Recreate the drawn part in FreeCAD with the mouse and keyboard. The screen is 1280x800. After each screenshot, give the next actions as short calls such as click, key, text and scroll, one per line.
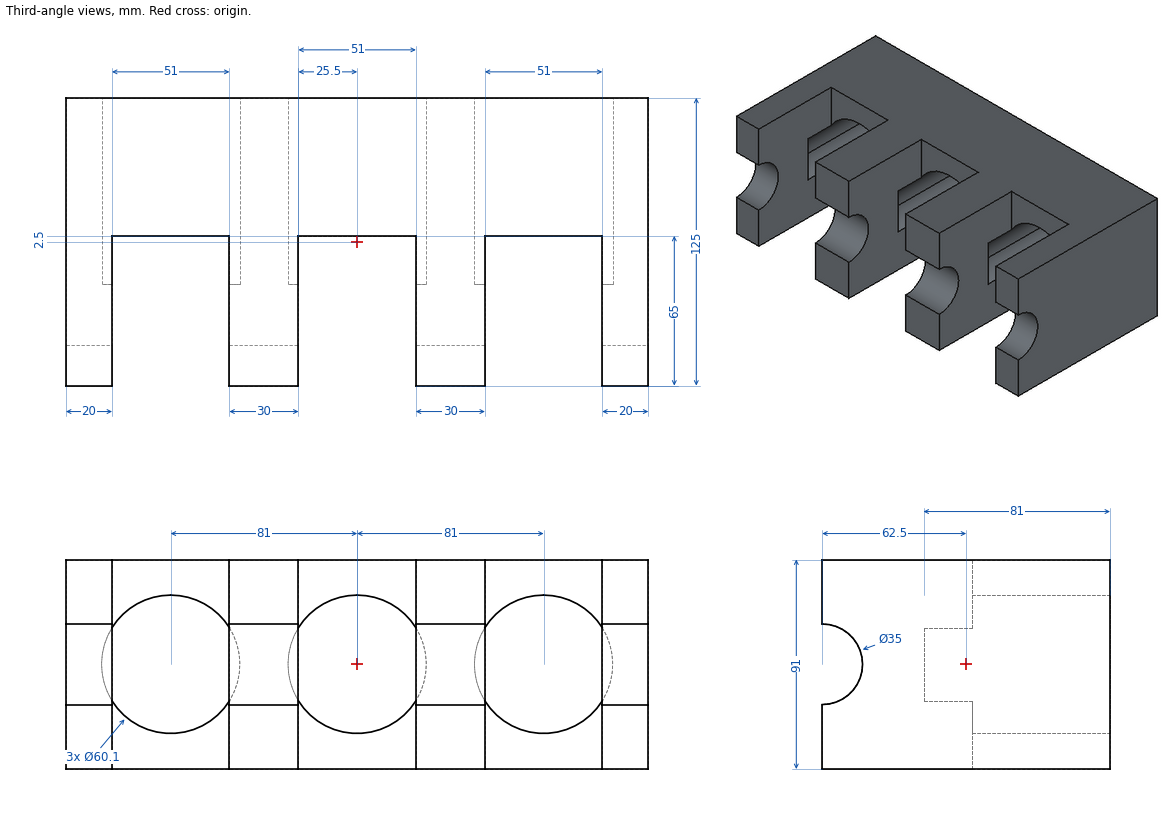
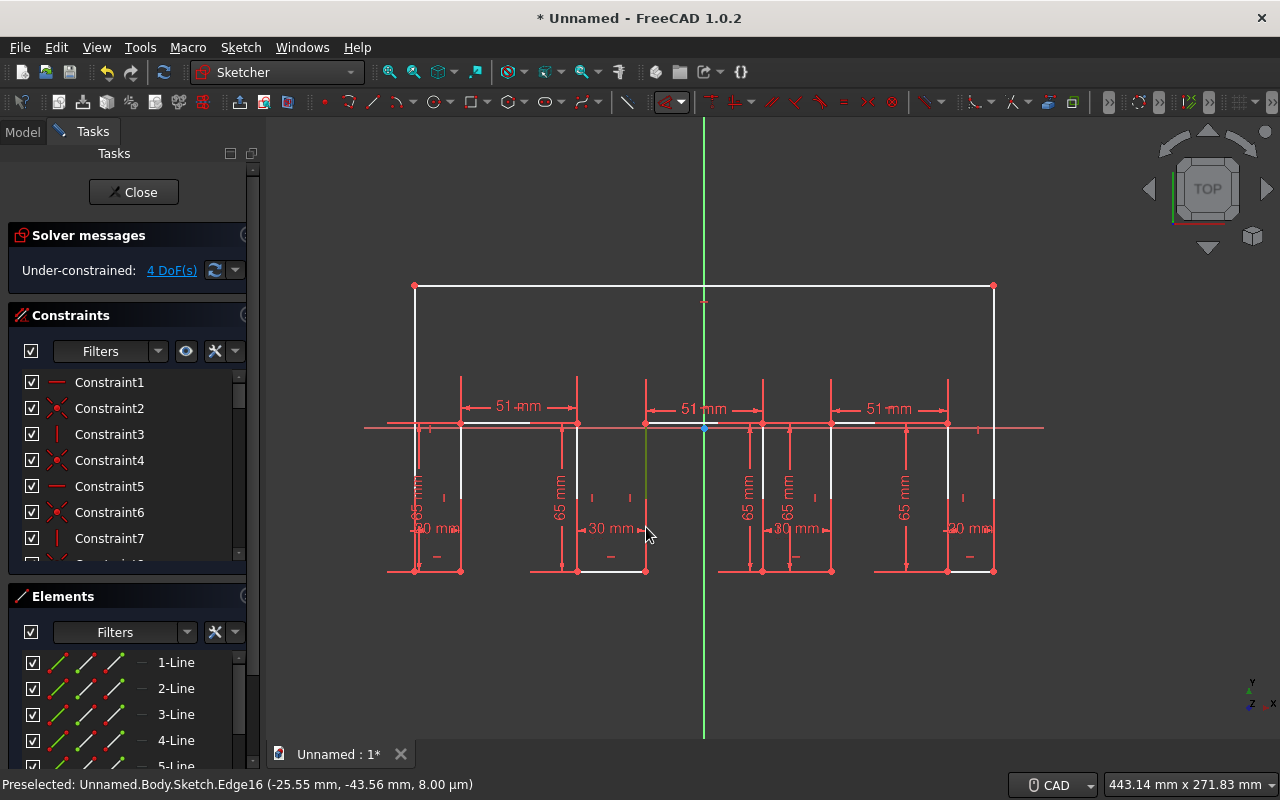
click(684, 102)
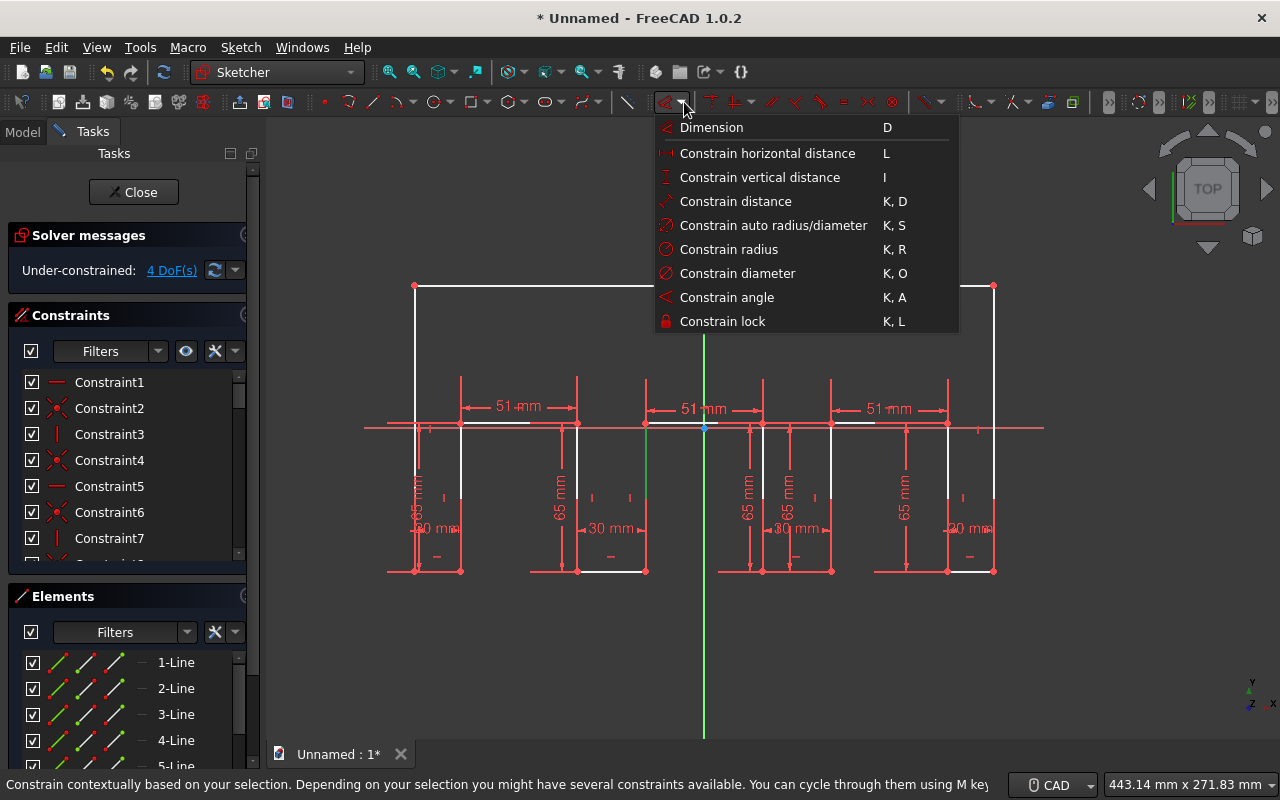
click(807, 177)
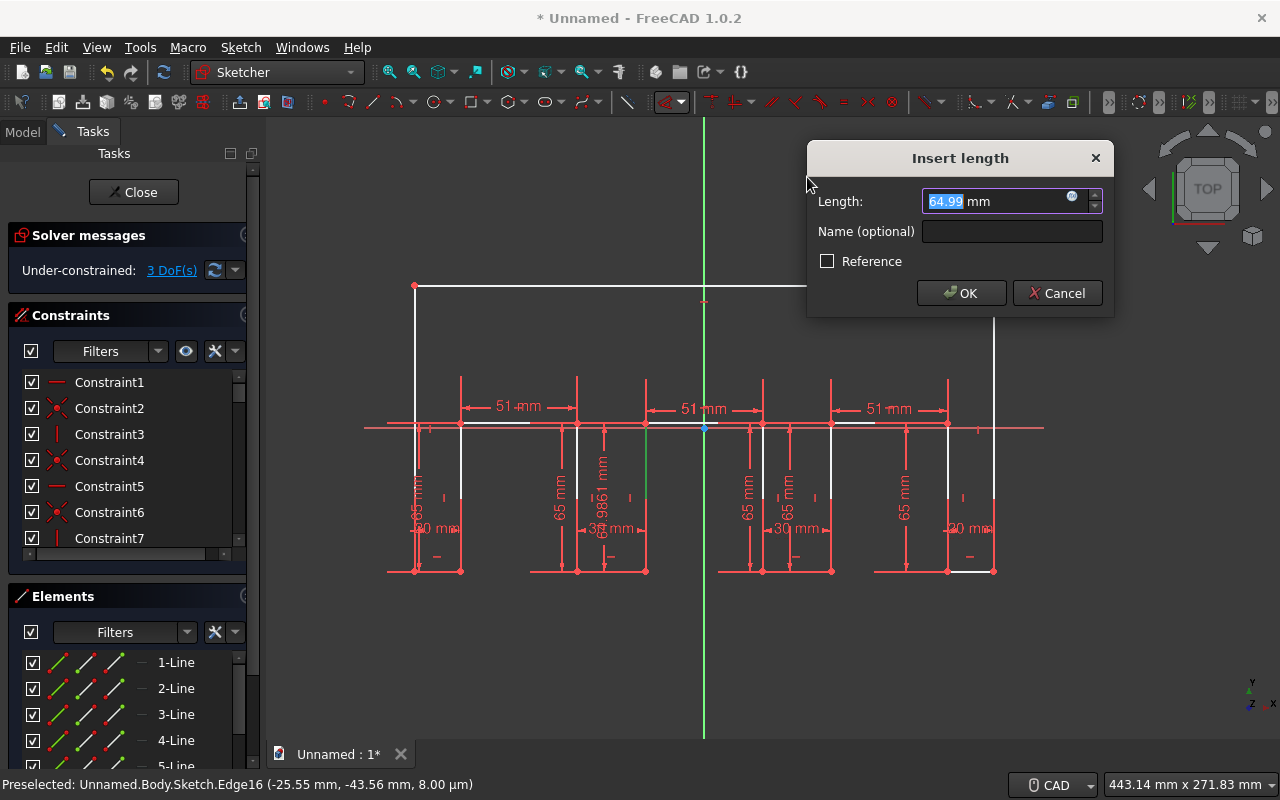
text(65)
key(Return)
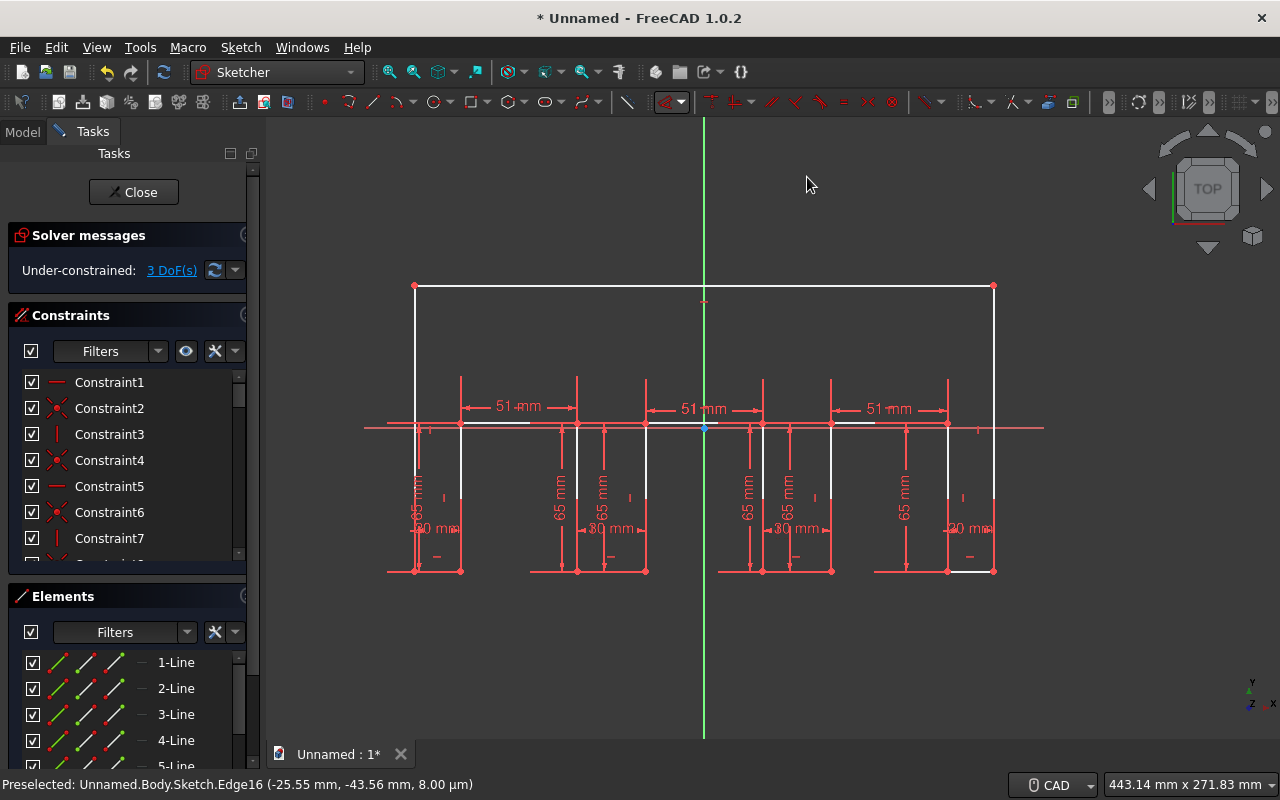
click(994, 486)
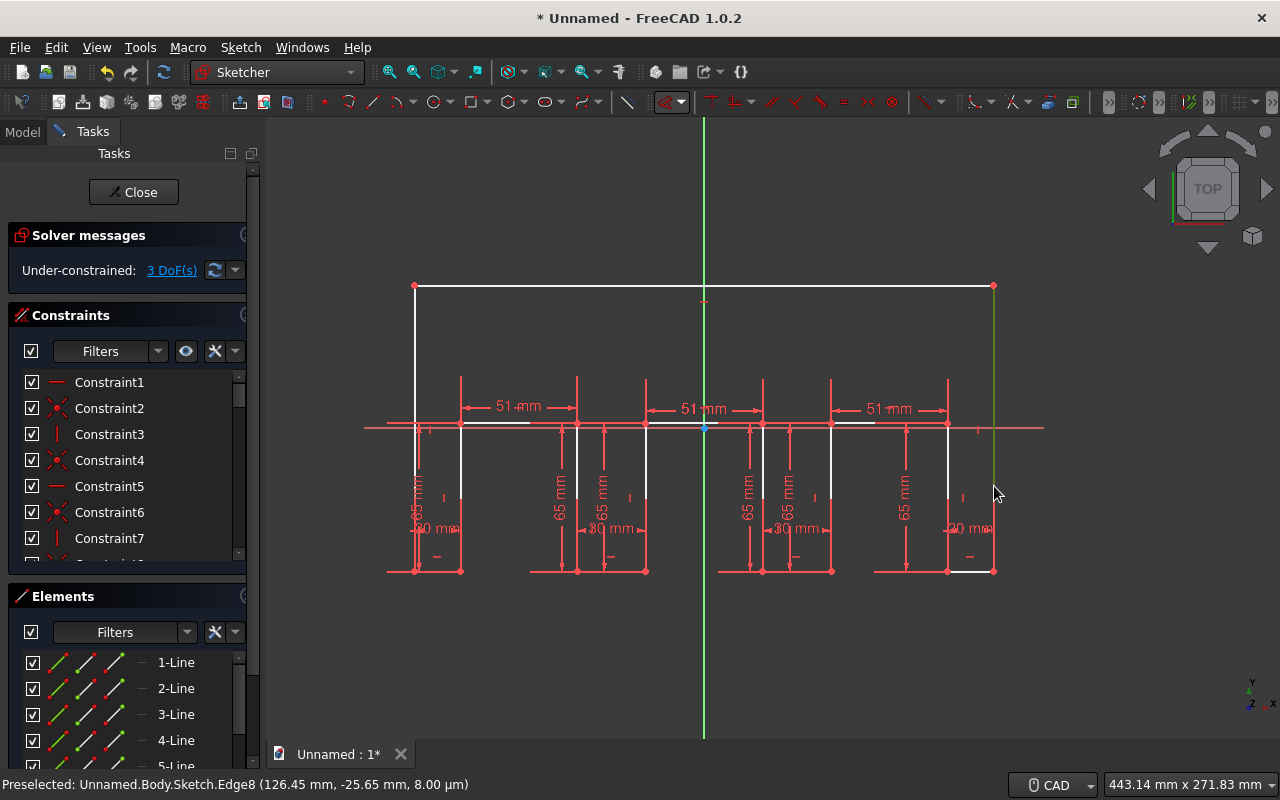
key(i)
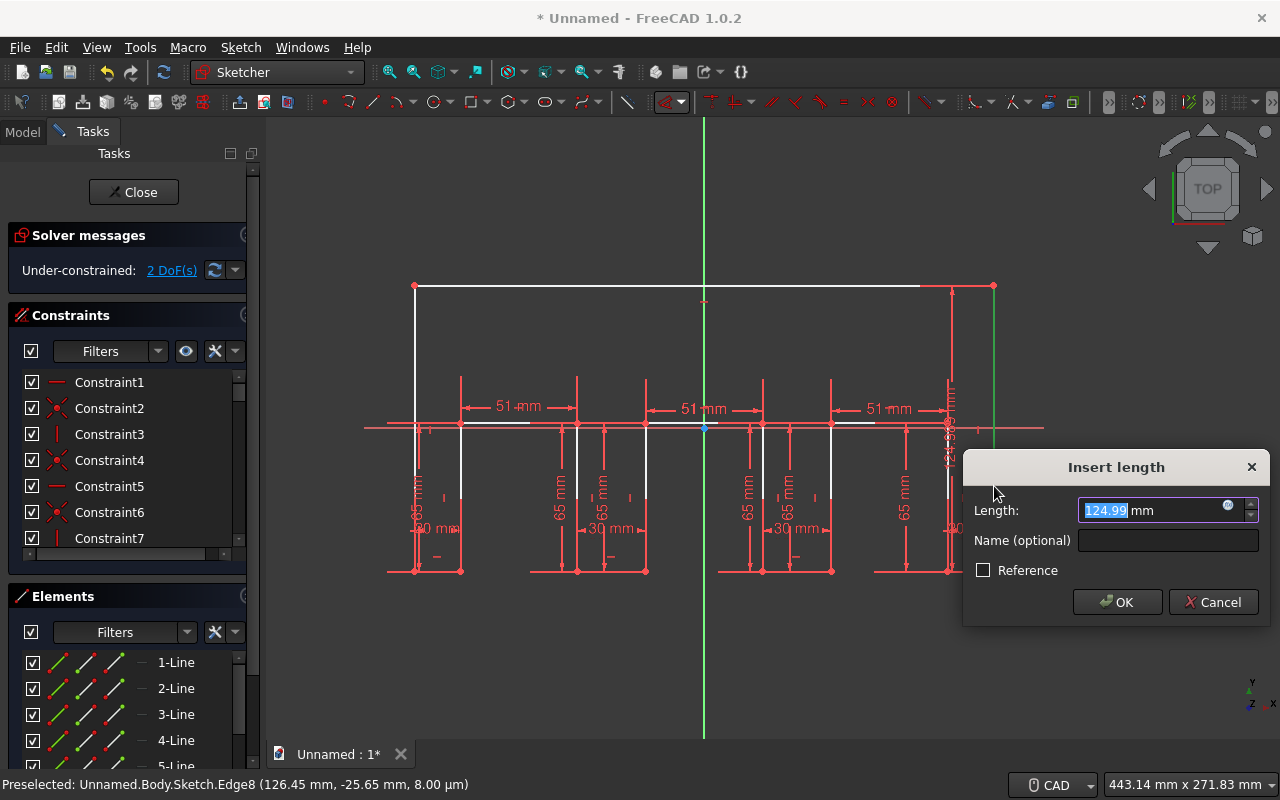
text(125)
key(Return)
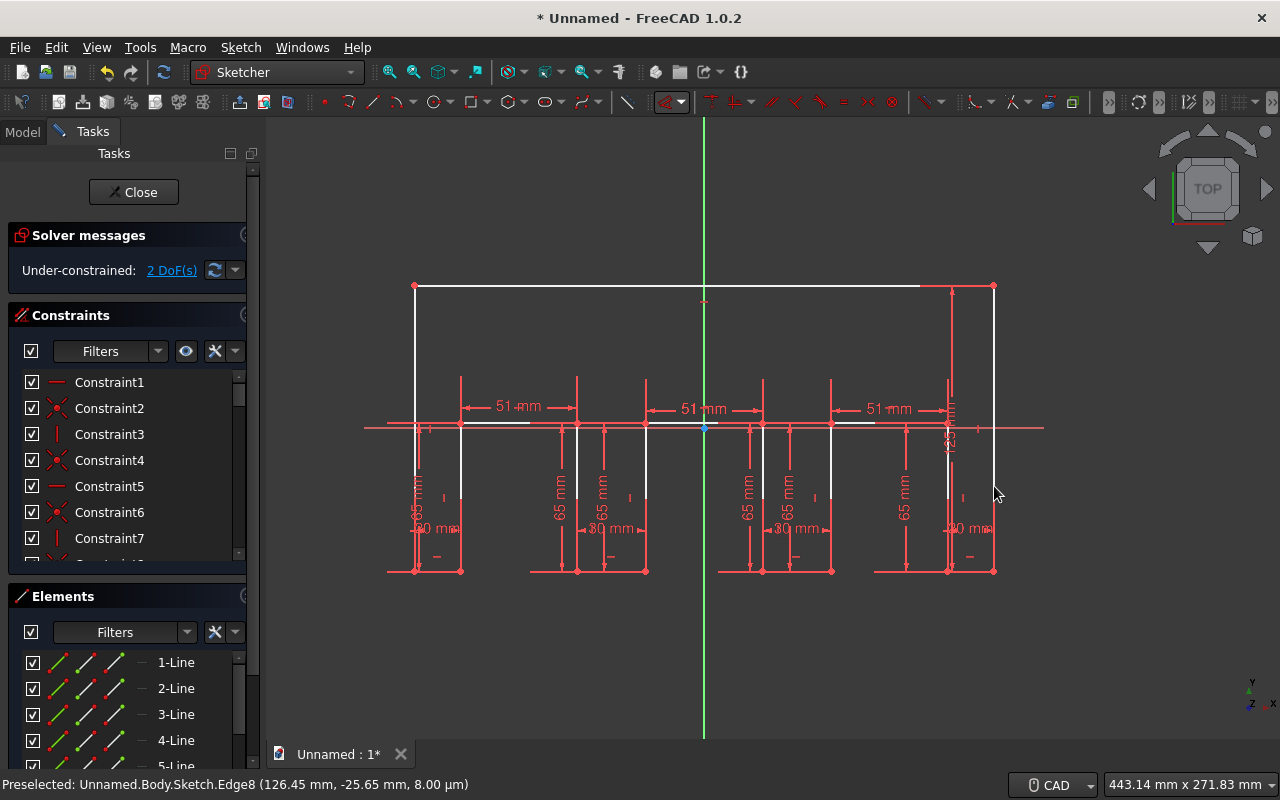
scroll(646, 423, up, 10)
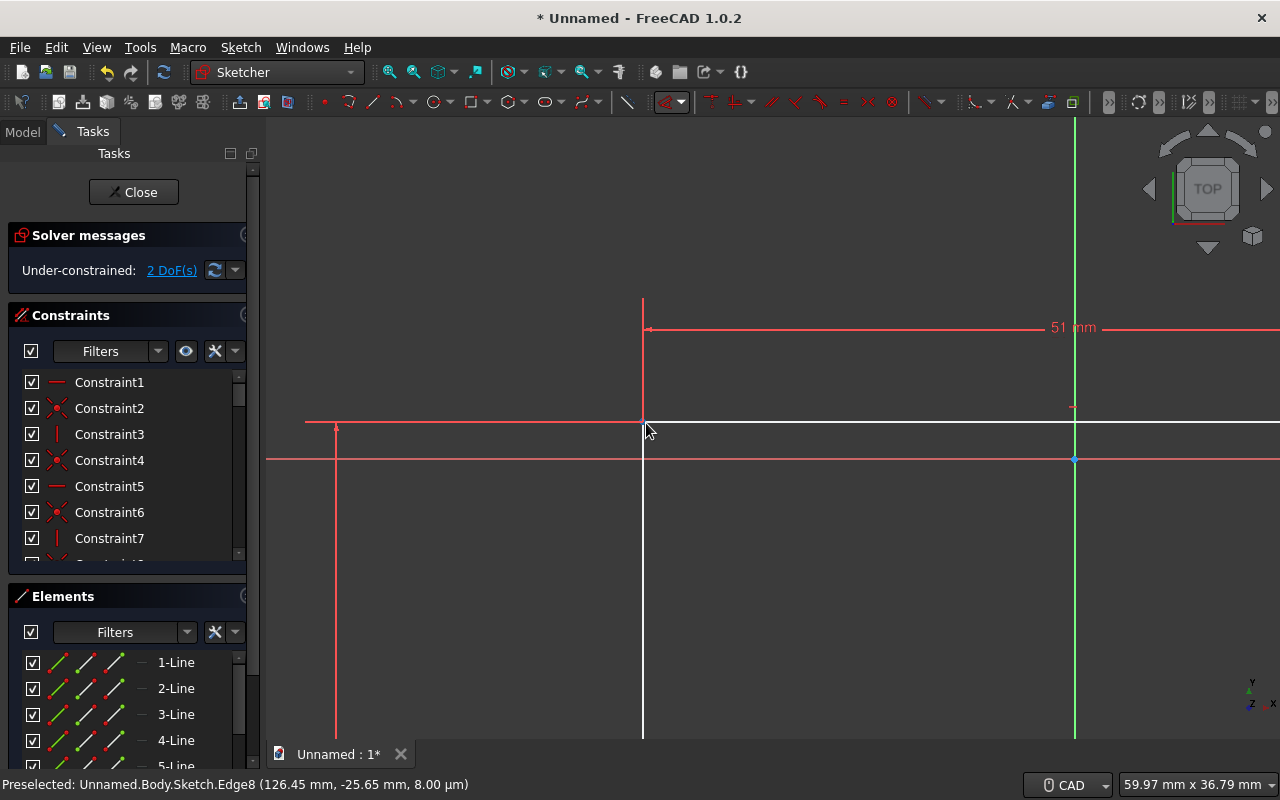
click(643, 422)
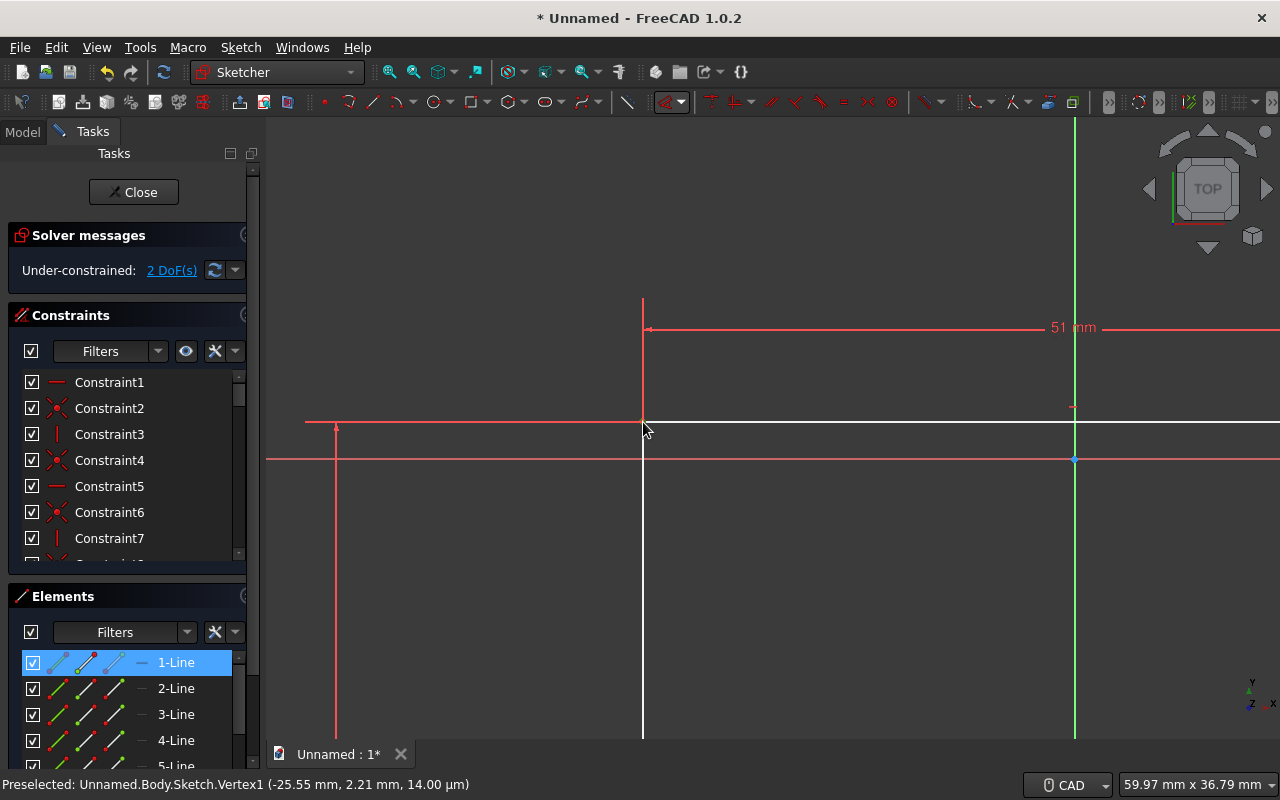
click(684, 102)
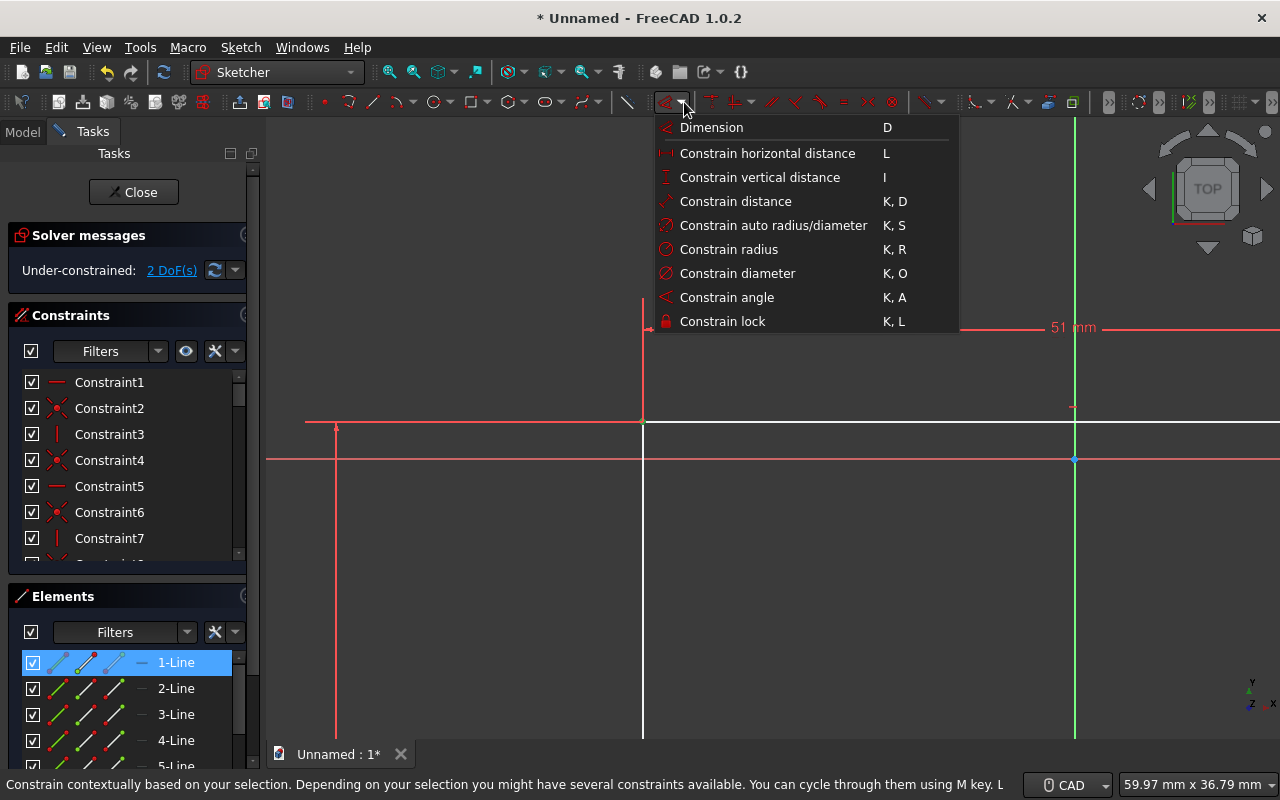
click(807, 177)